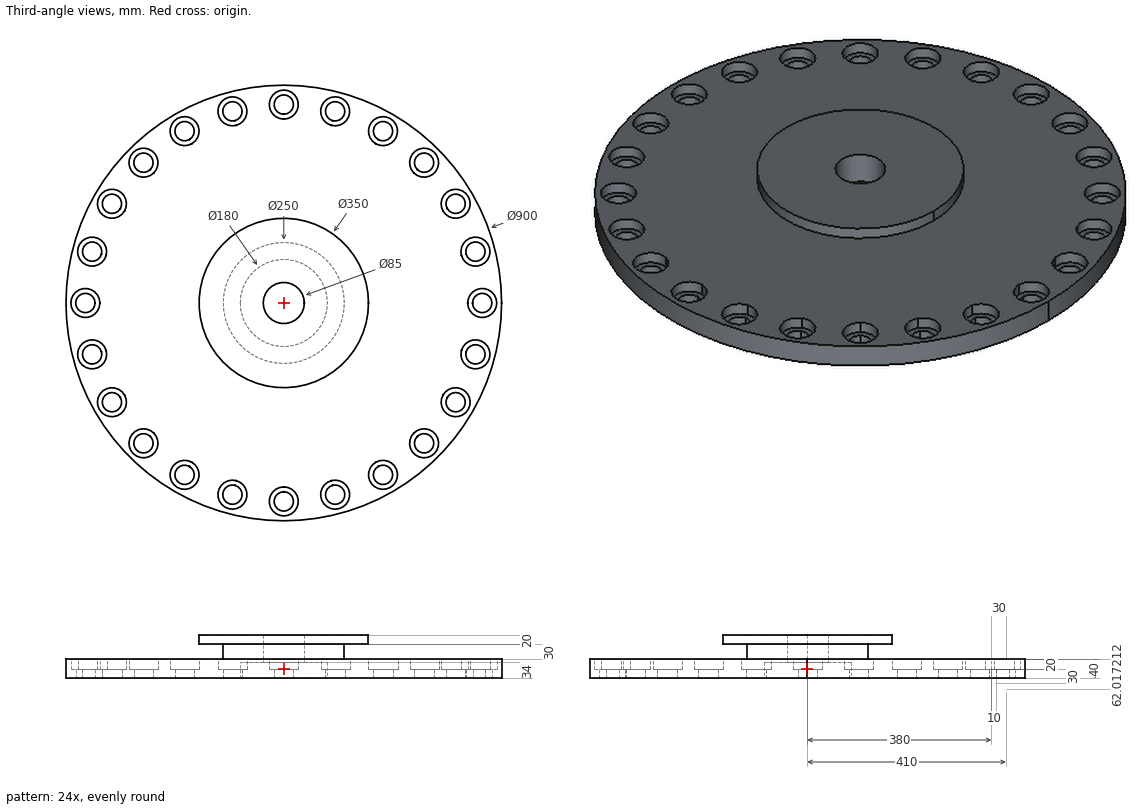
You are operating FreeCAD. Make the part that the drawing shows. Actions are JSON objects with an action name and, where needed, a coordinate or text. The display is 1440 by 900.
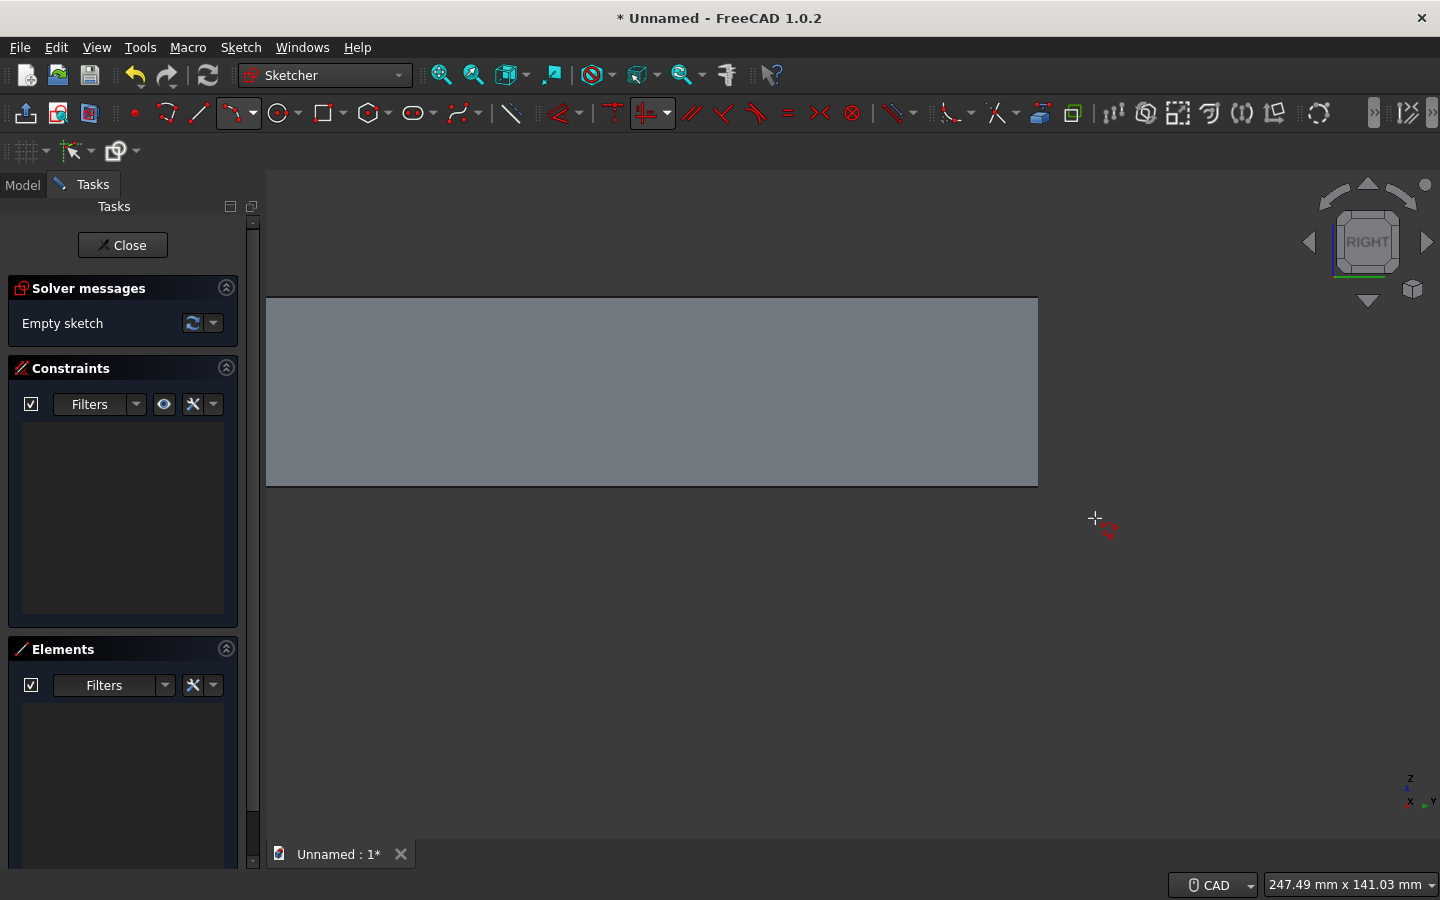
{"action": "left_click", "coordinate": [708, 392]}
{"action": "left_click", "coordinate": [755, 401]}
{"action": "left_click", "coordinate": [755, 534]}
{"action": "left_click", "coordinate": [850, 591]}
{"action": "left_click", "coordinate": [850, 297]}
{"action": "left_click", "coordinate": [708, 297]}
{"action": "left_click", "coordinate": [708, 393]}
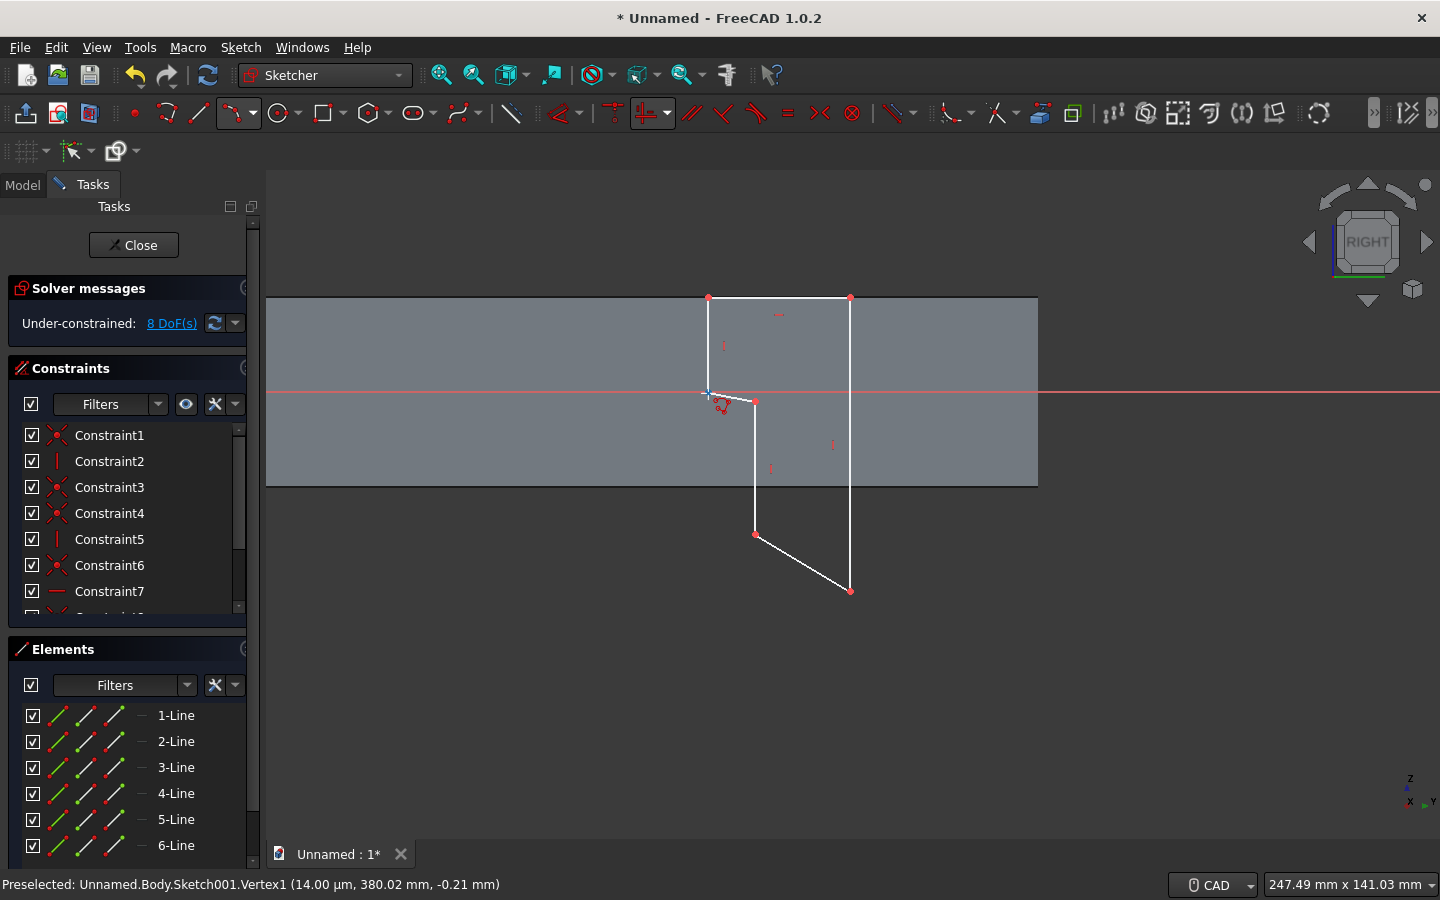
{"action": "key", "text": "g l"}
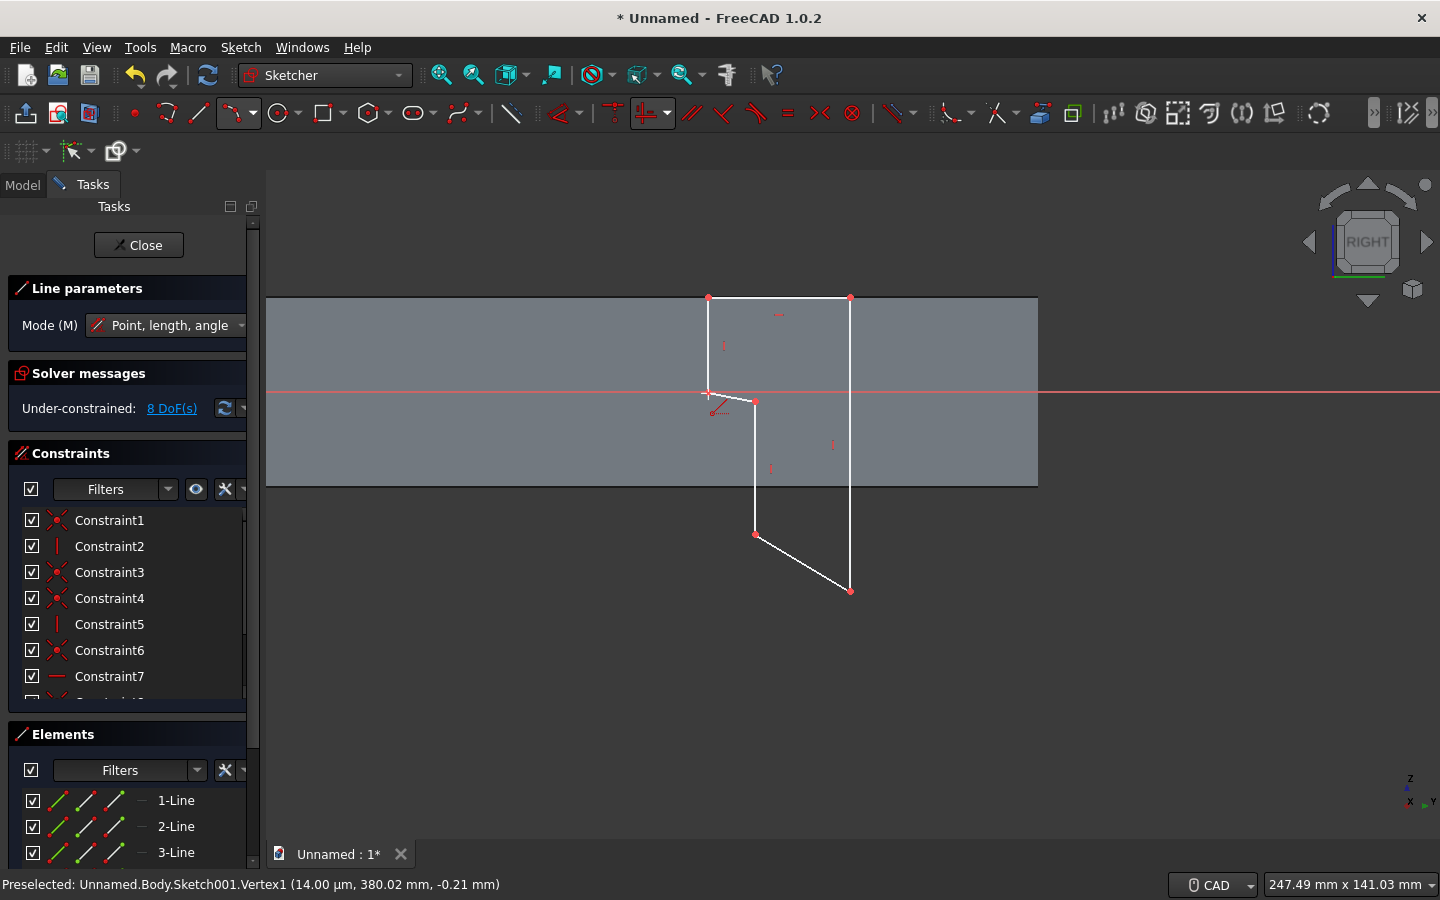
{"action": "left_click", "coordinate": [850, 621]}
{"action": "left_click", "coordinate": [850, 709]}
{"action": "key", "text": "Escape"}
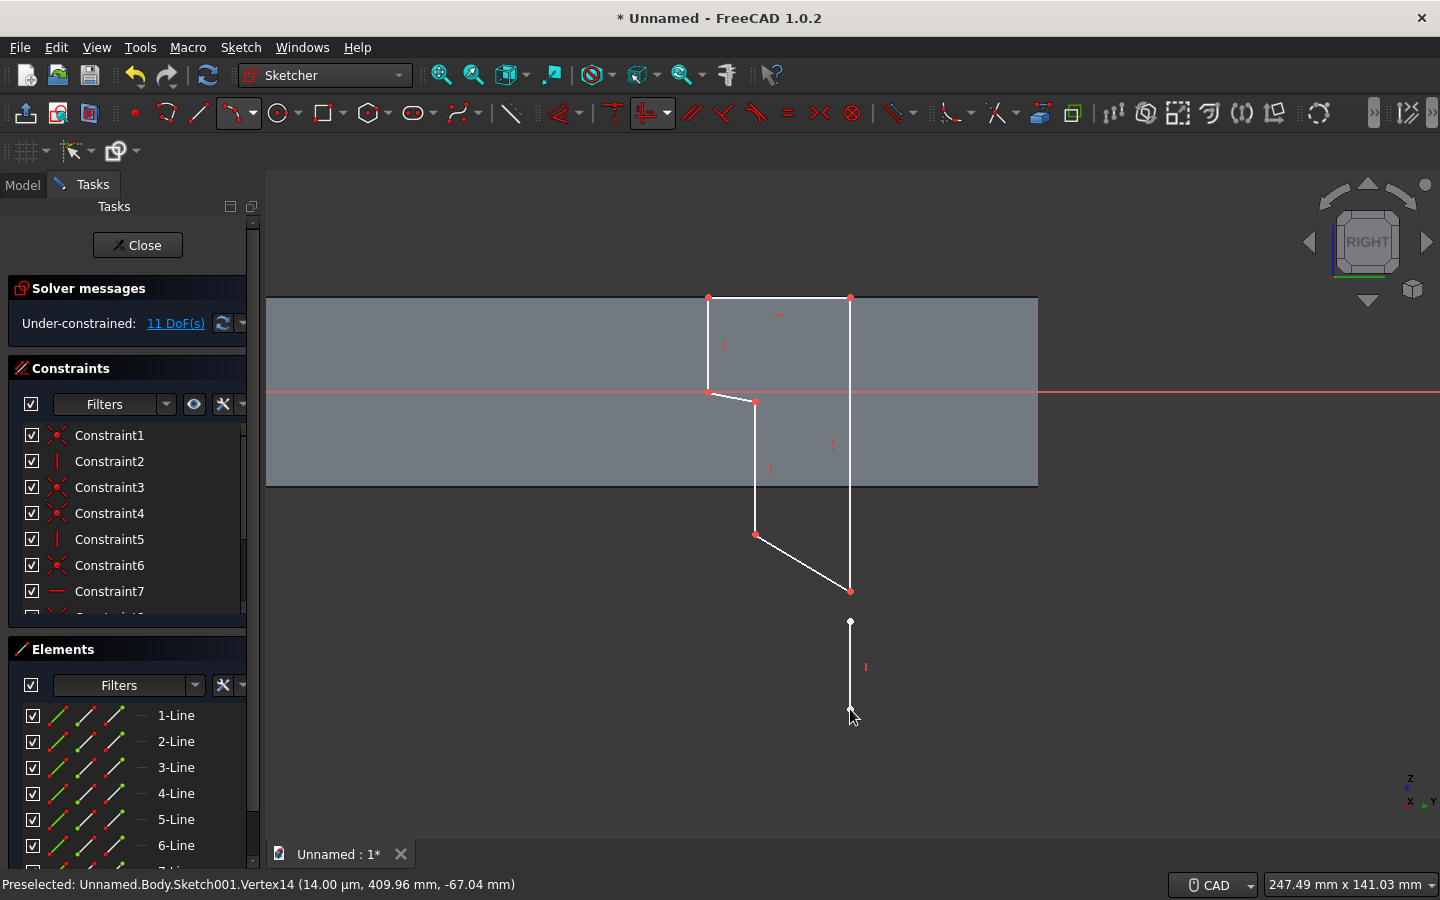
{"action": "left_click", "coordinate": [850, 648]}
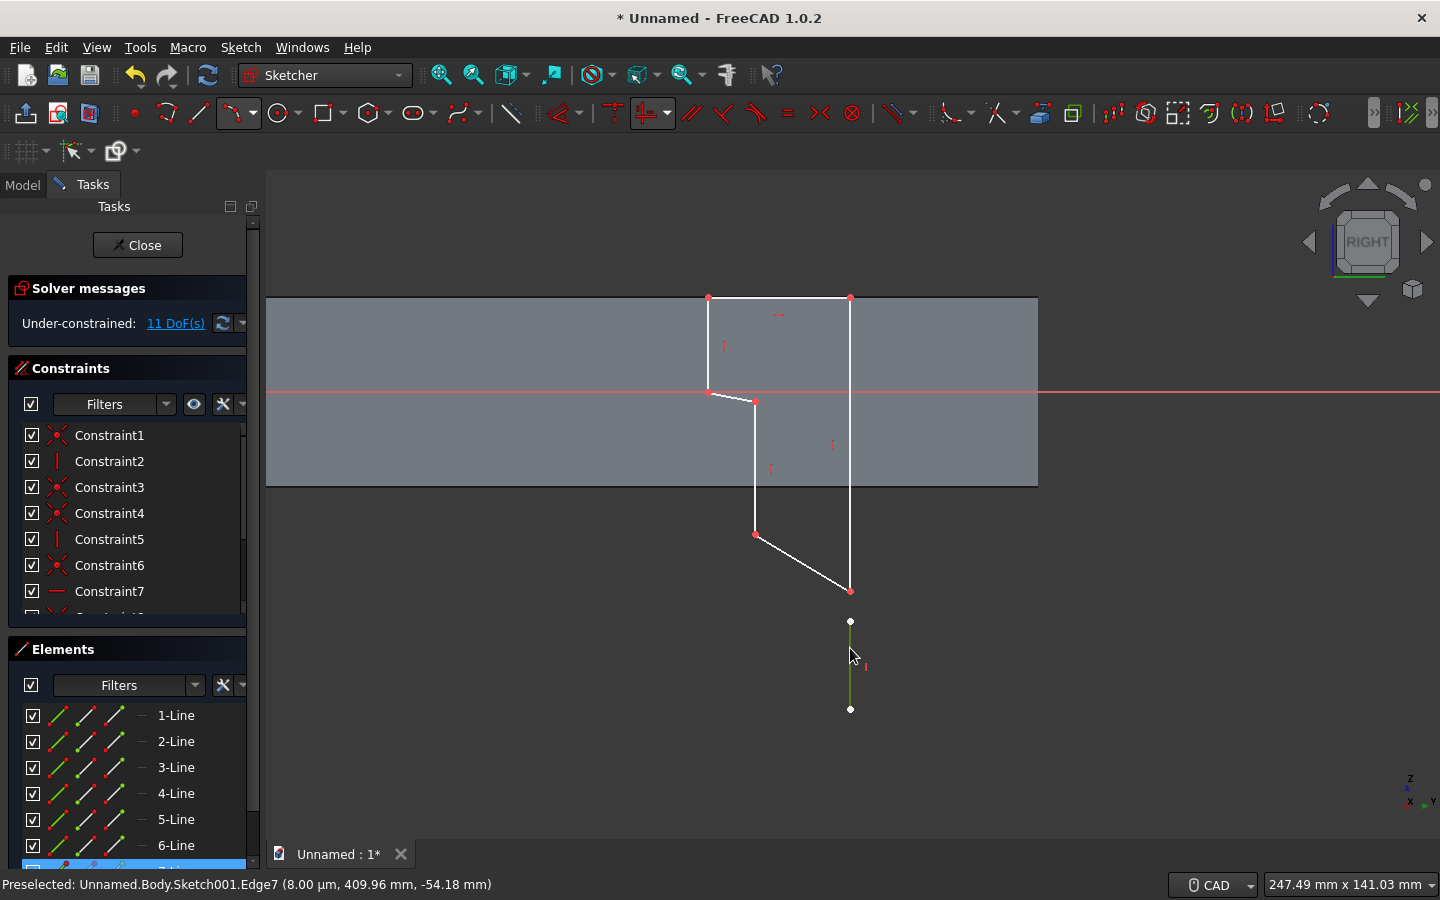
{"action": "left_click", "coordinate": [512, 114]}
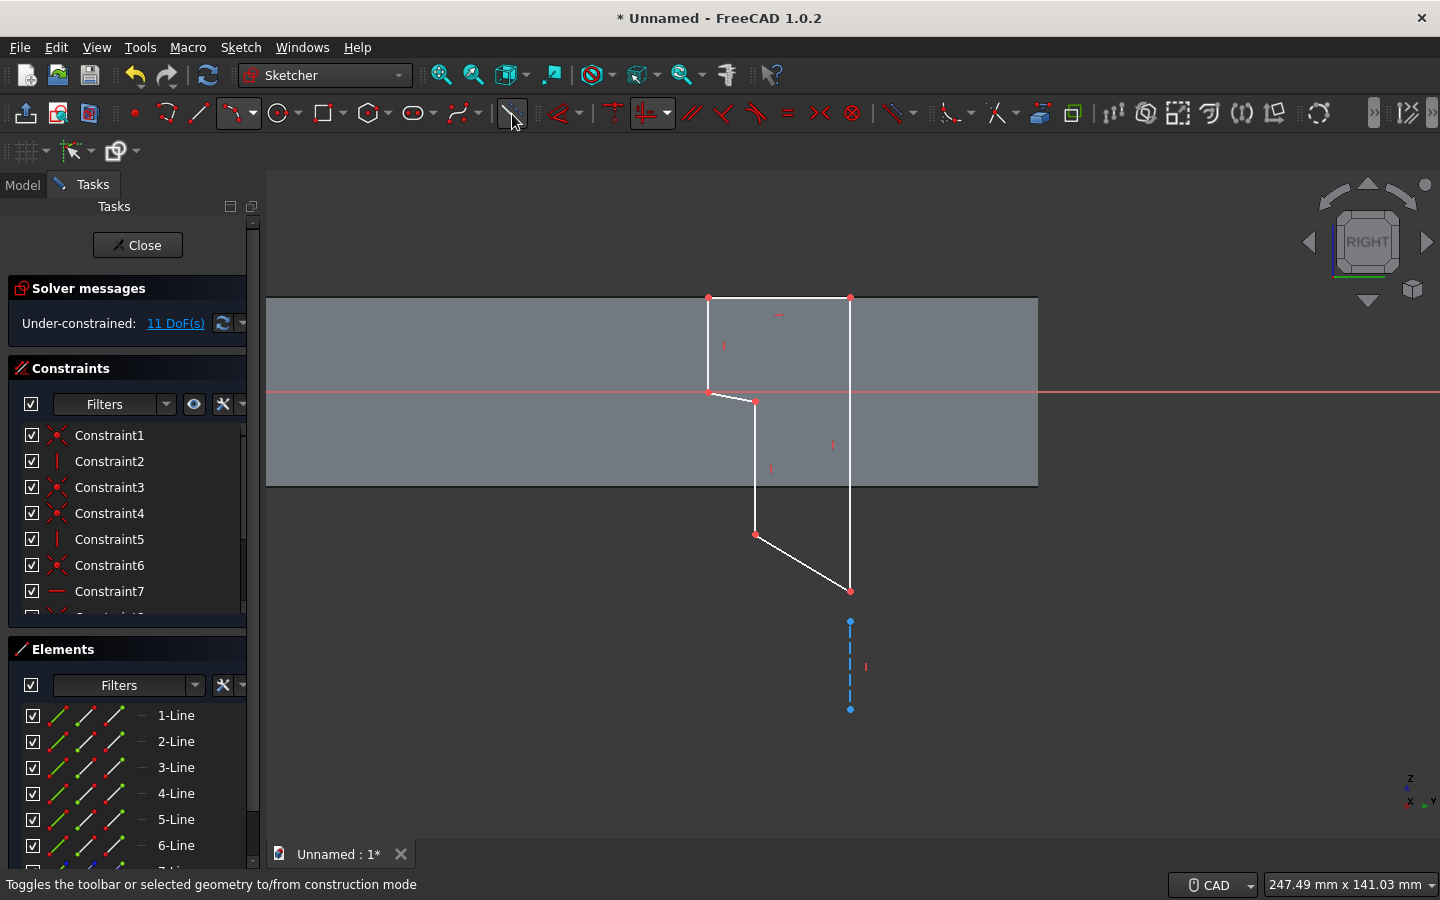
{"action": "left_click", "coordinate": [722, 396]}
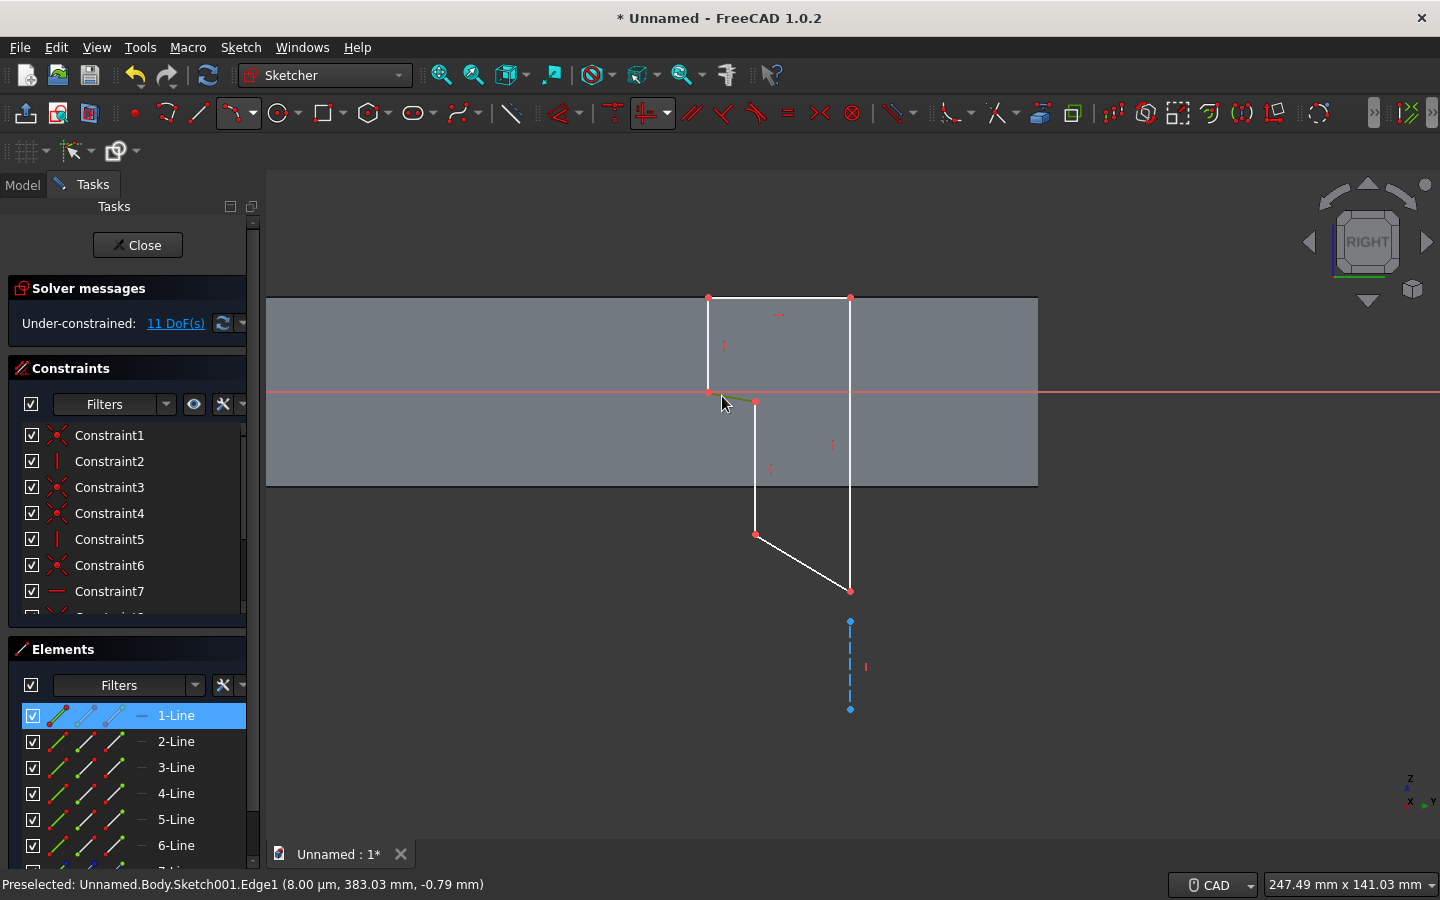
{"action": "left_click", "coordinate": [670, 114]}